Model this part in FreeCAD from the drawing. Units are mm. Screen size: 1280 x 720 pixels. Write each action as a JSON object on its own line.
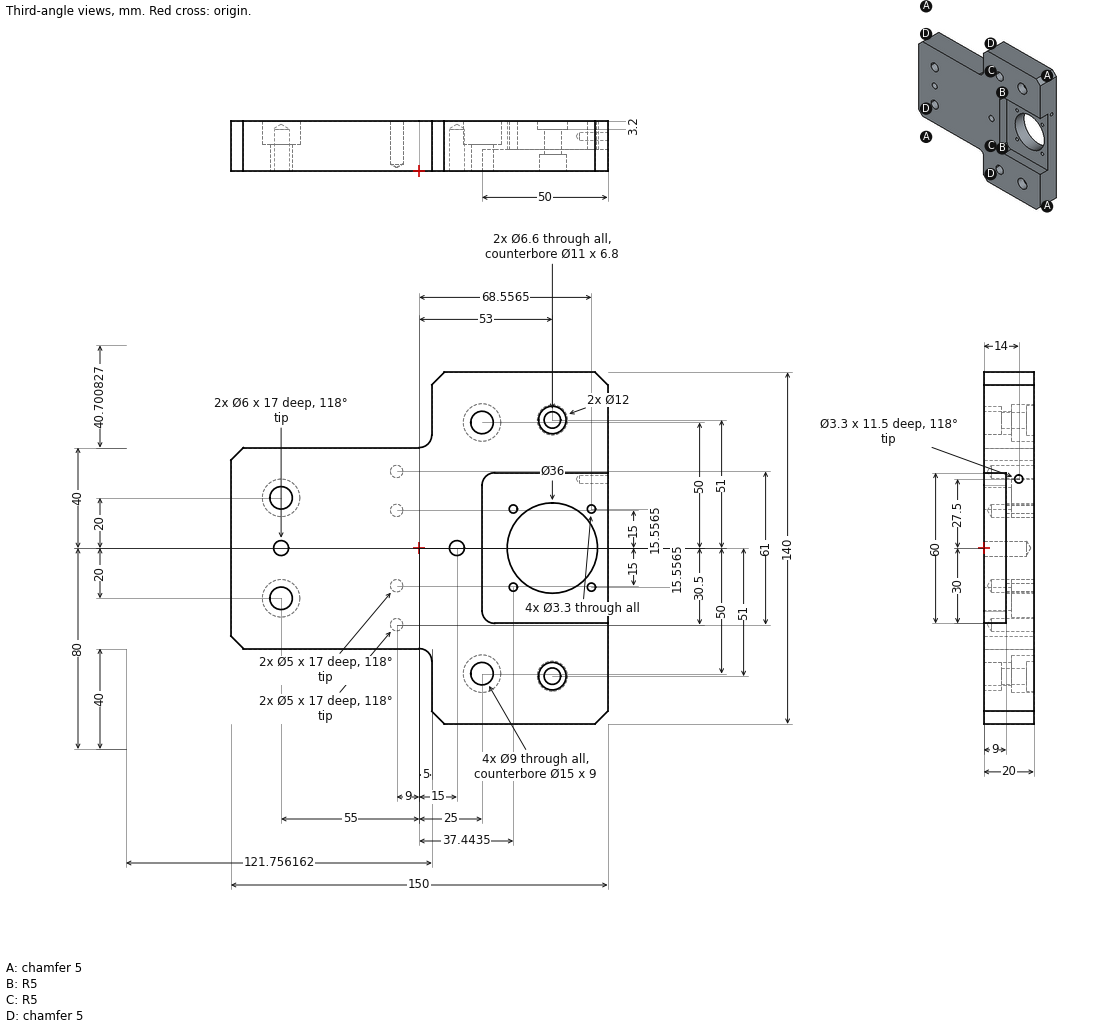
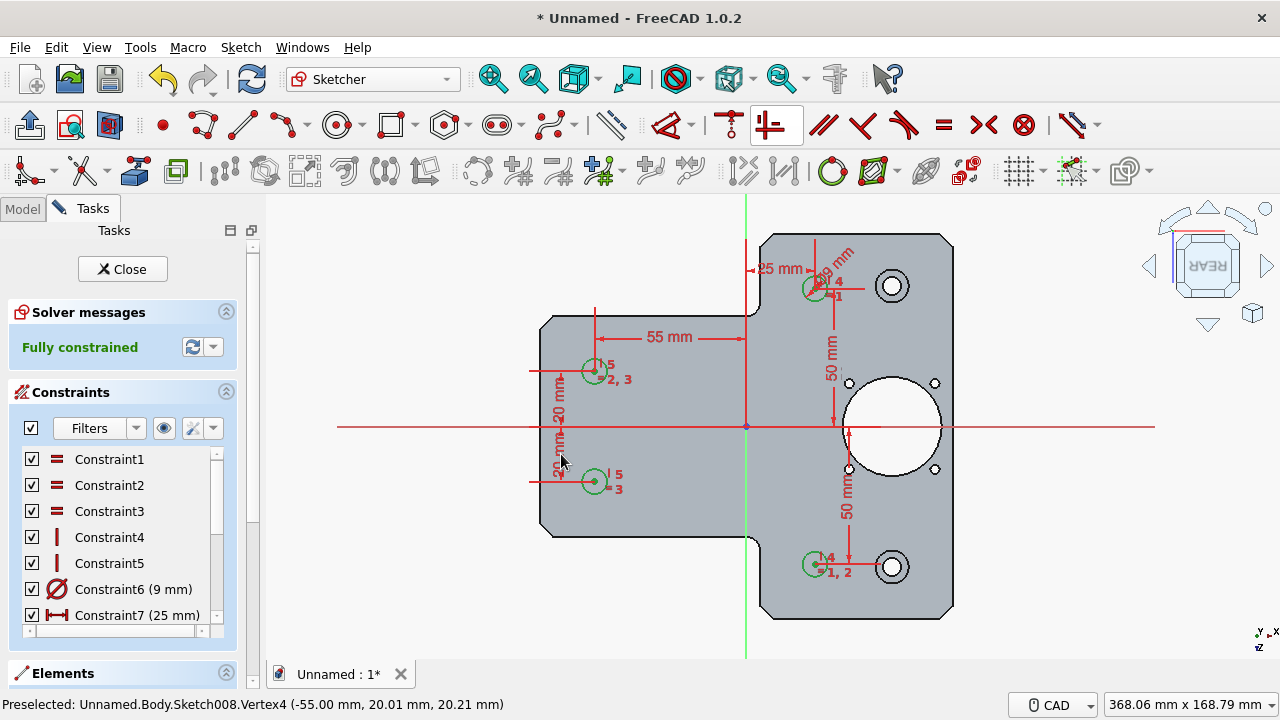
{"action": "left_click", "coordinate": [123, 269]}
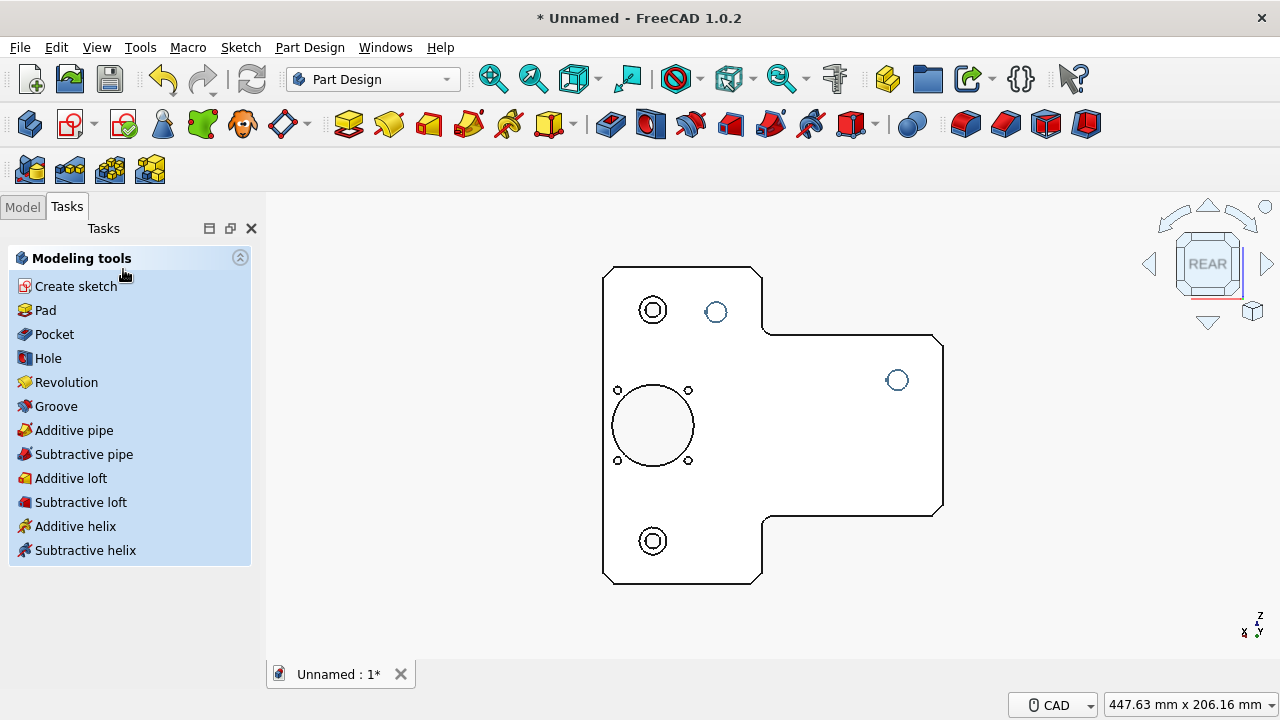
{"action": "left_click", "coordinate": [652, 124]}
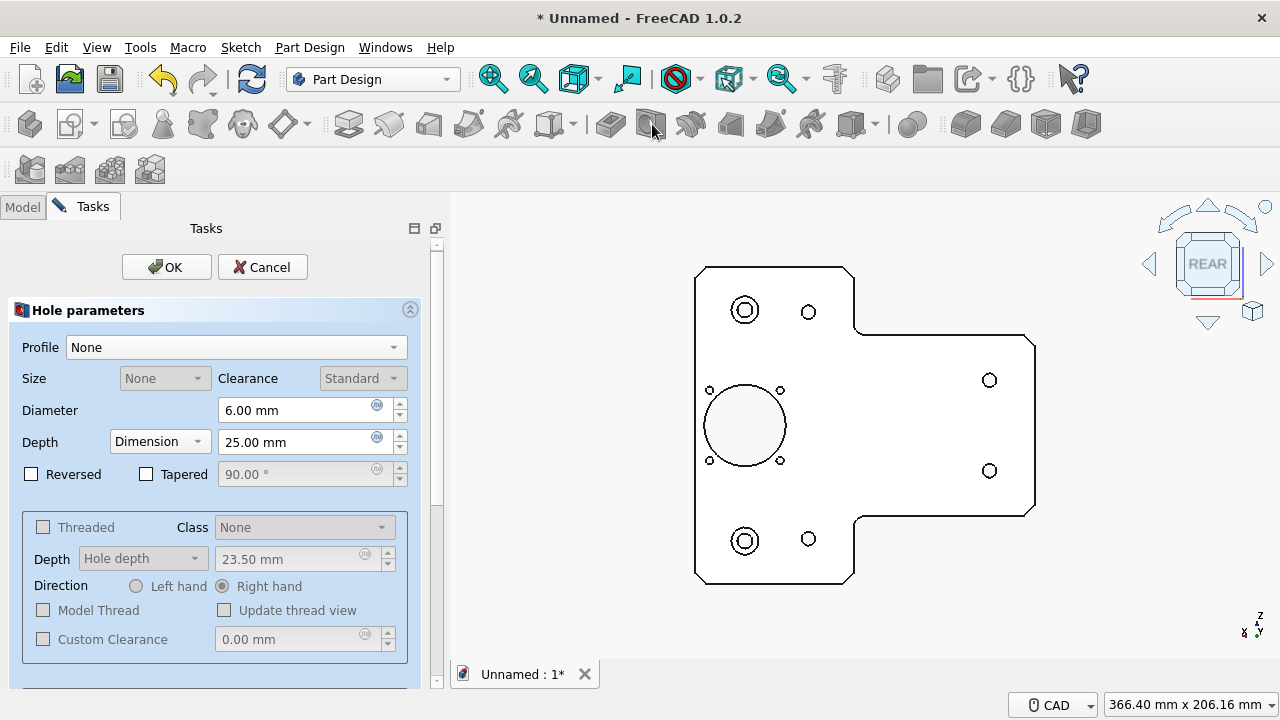
{"action": "triple_click", "coordinate": [305, 410]}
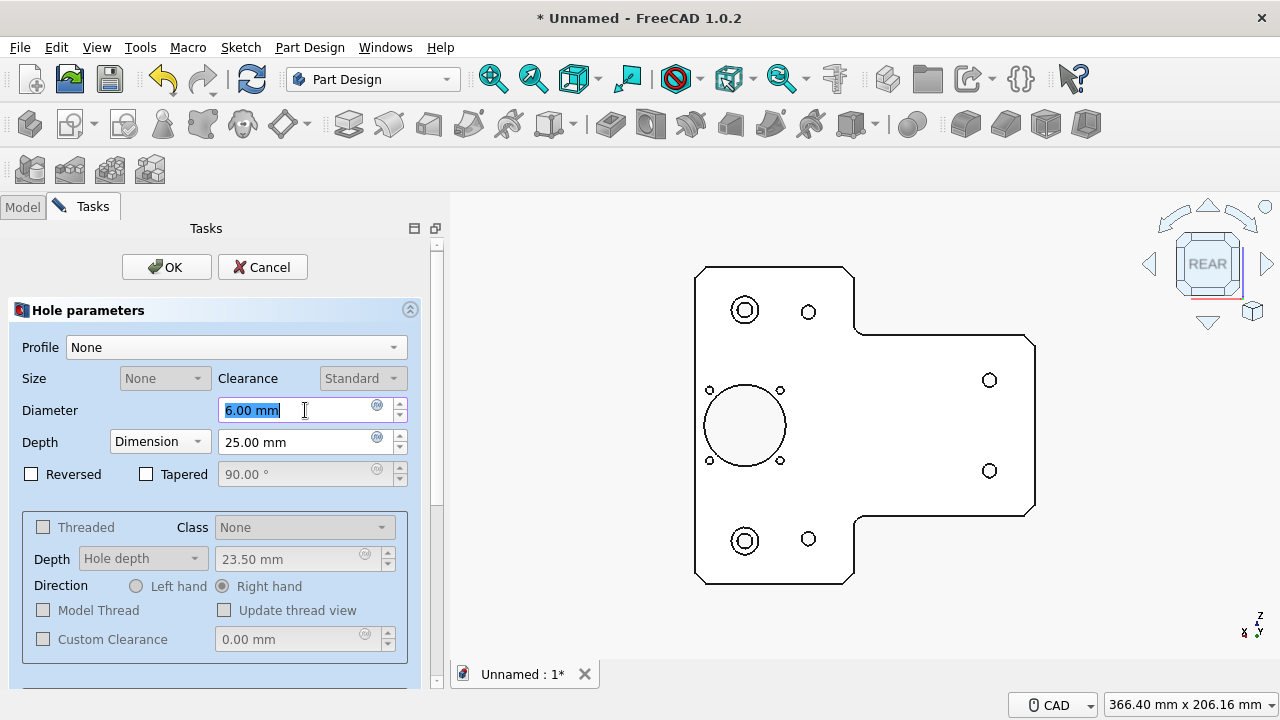
{"action": "type", "text": "9"}
{"action": "key", "text": "Tab"}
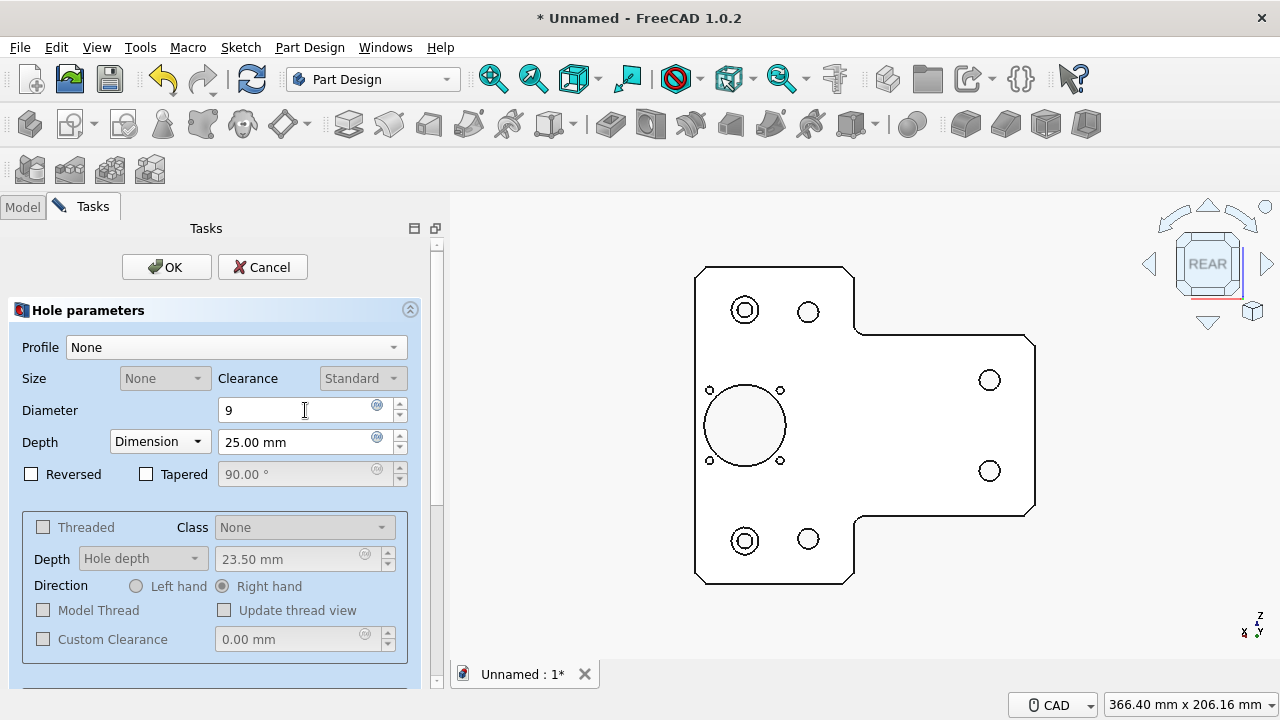
{"action": "left_click", "coordinate": [161, 442]}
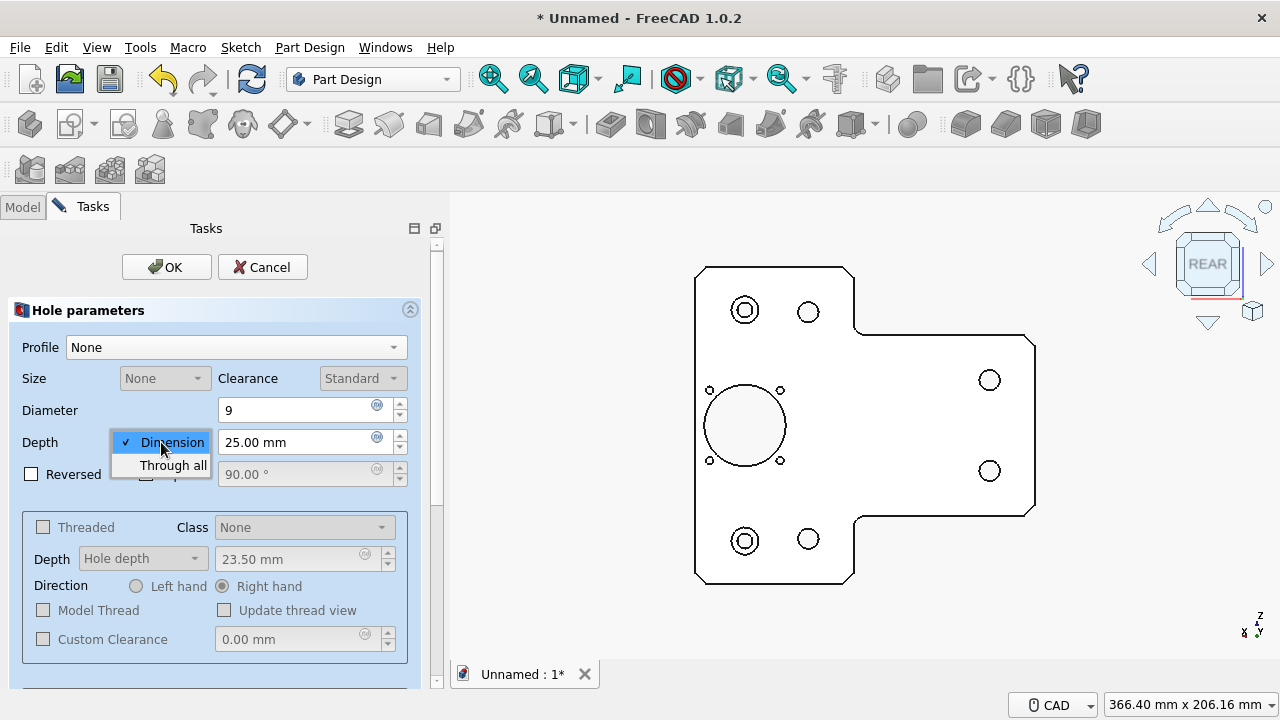
{"action": "left_click", "coordinate": [160, 466]}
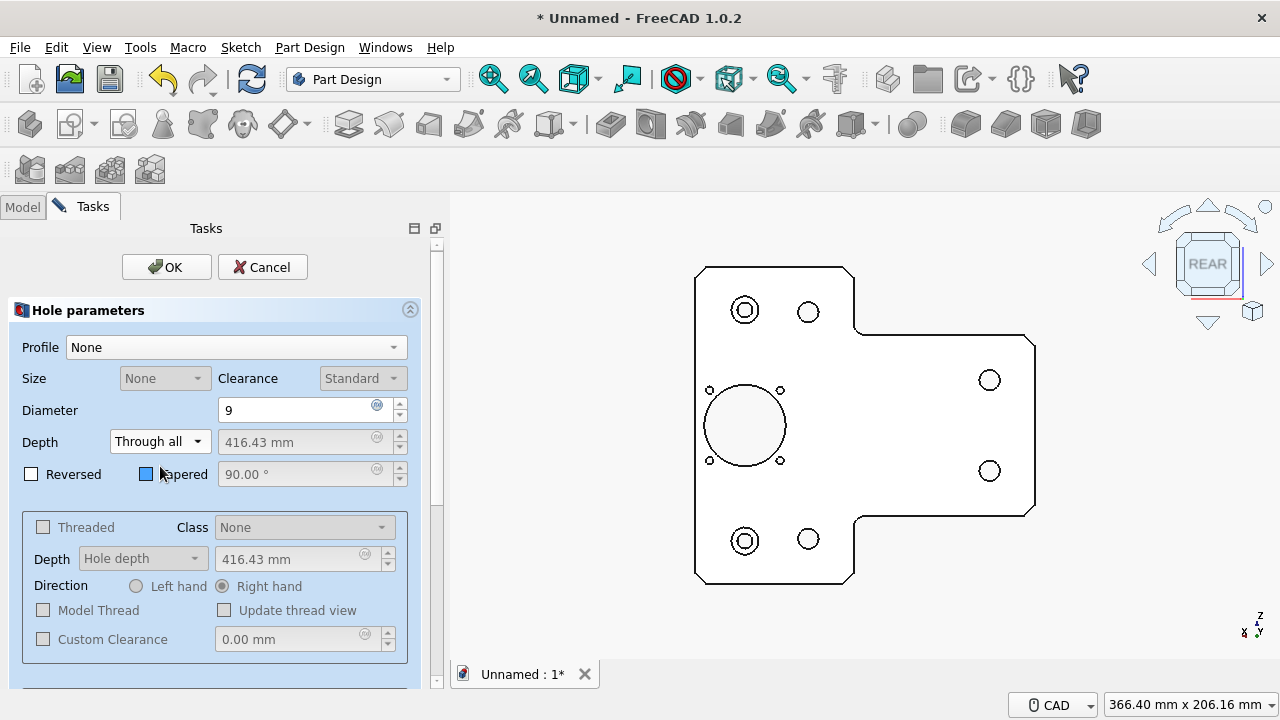
{"action": "scroll", "coordinate": [437, 463], "scroll_direction": "down", "scroll_amount": 2}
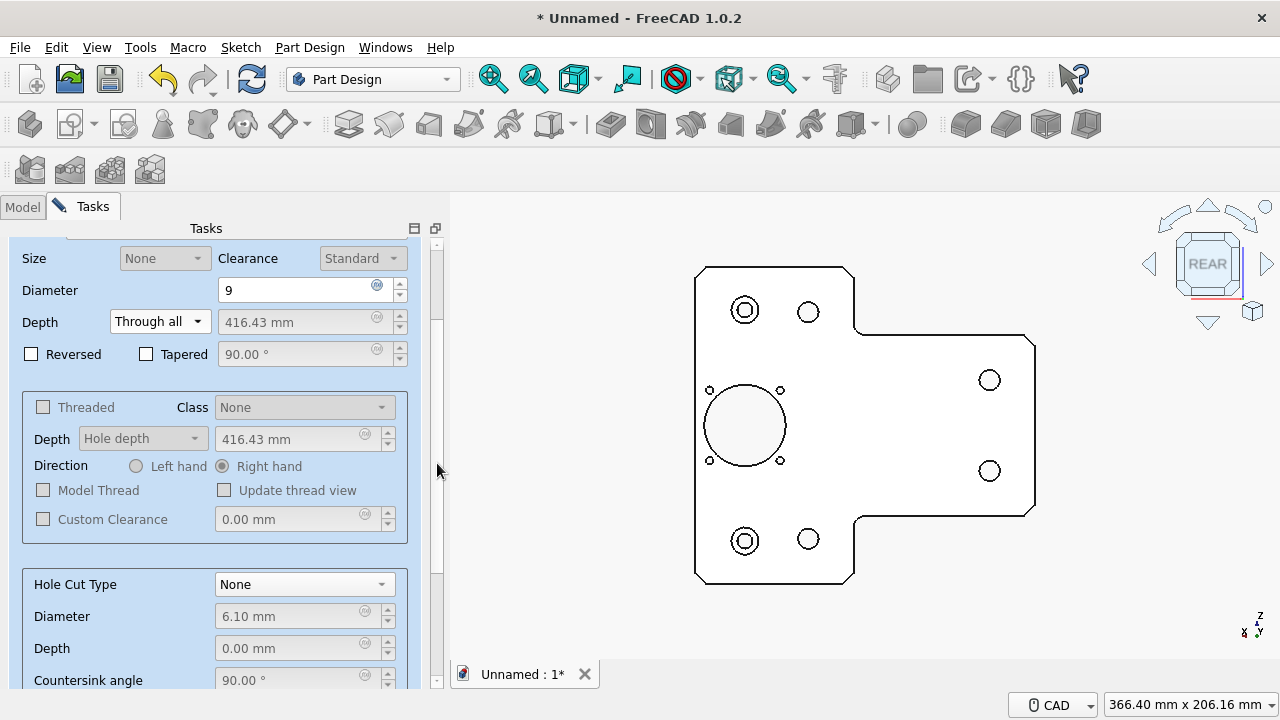
{"action": "left_click", "coordinate": [306, 584]}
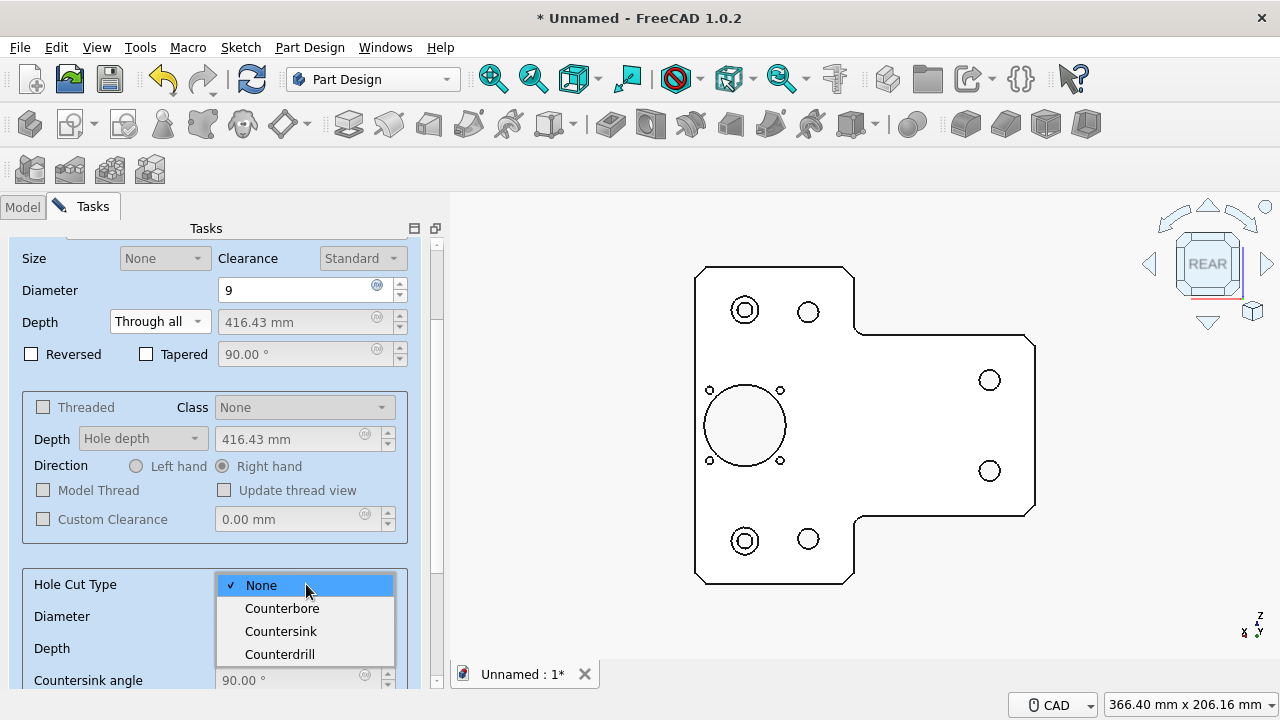
{"action": "left_click", "coordinate": [304, 608]}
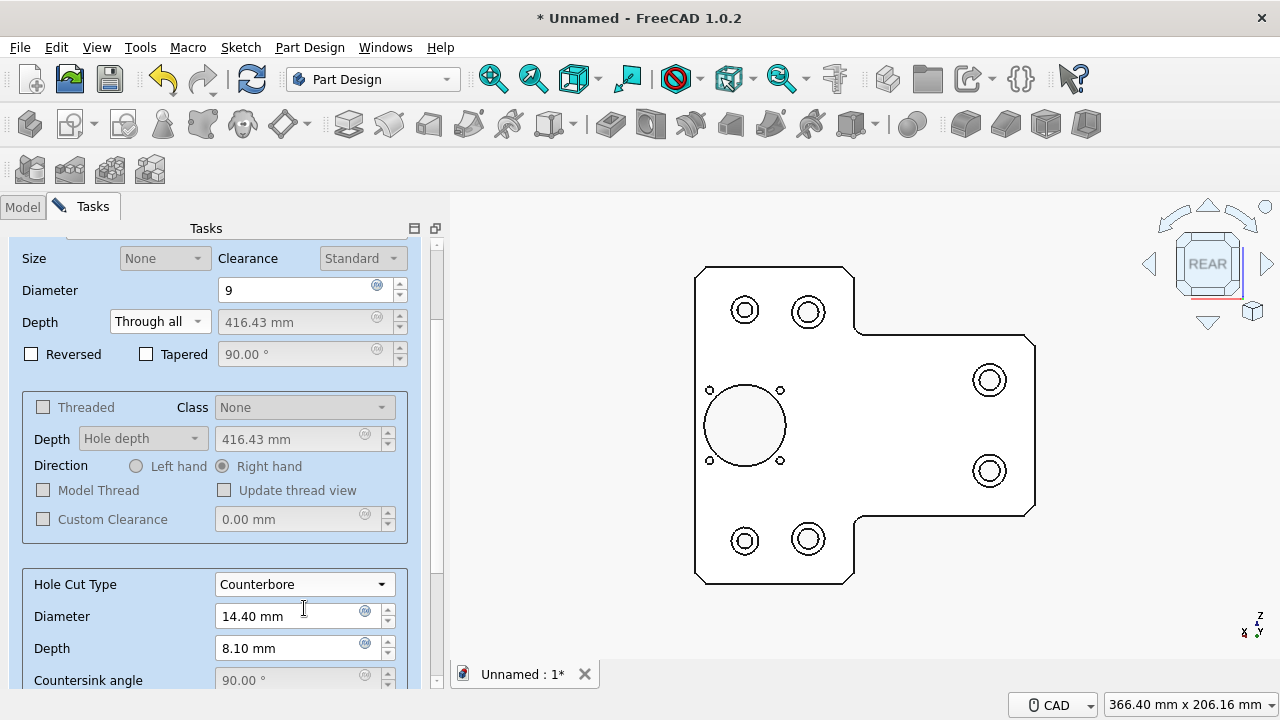
{"action": "triple_click", "coordinate": [298, 616]}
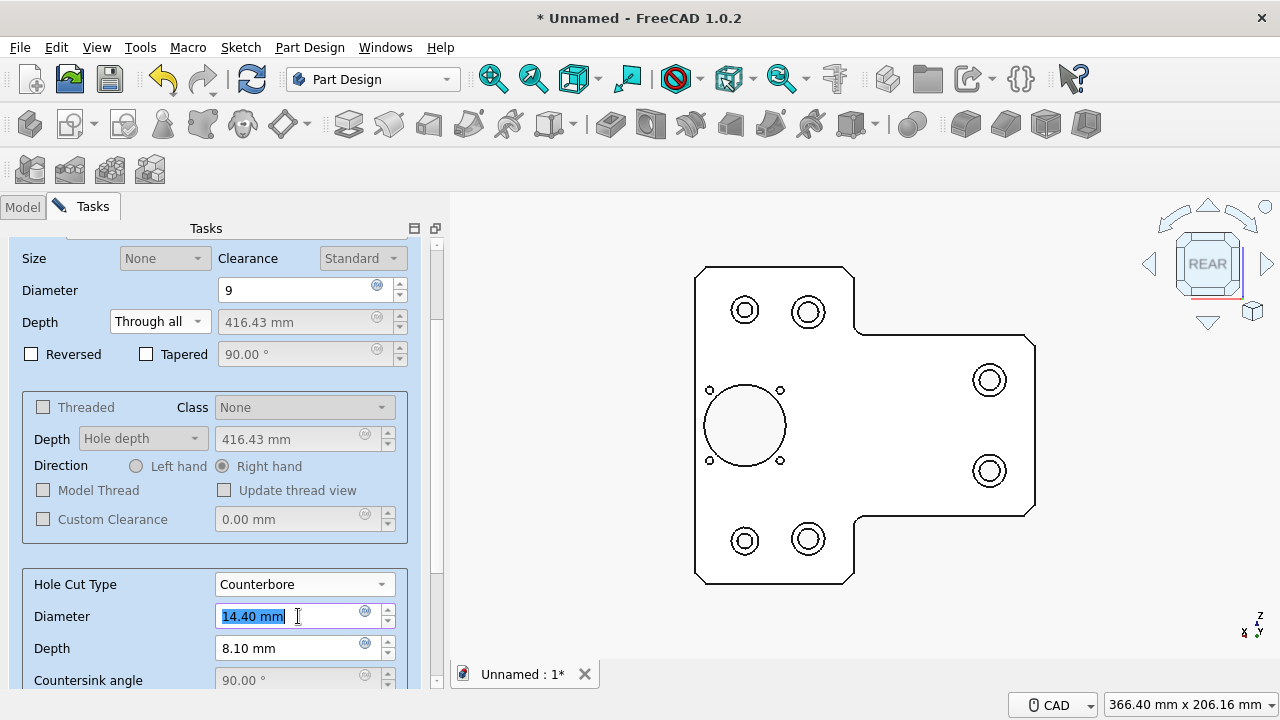
{"action": "type", "text": "15"}
{"action": "key", "text": "Tab"}